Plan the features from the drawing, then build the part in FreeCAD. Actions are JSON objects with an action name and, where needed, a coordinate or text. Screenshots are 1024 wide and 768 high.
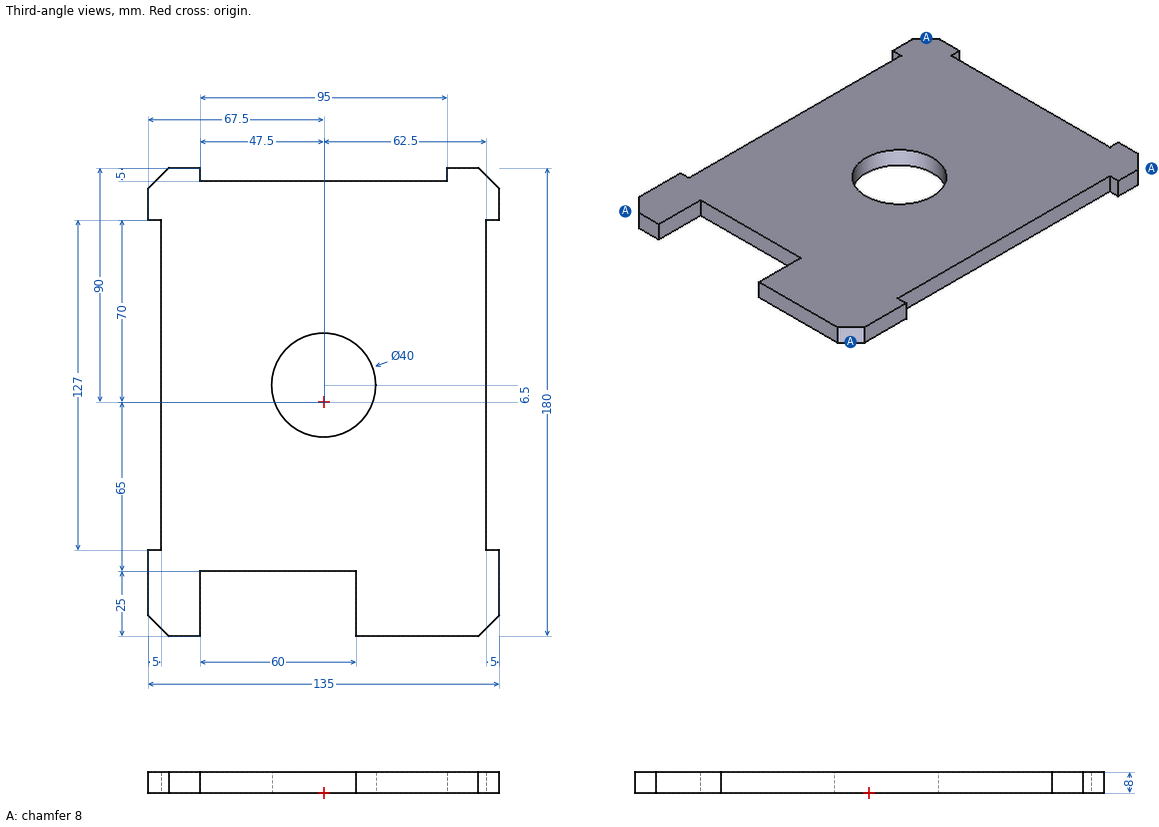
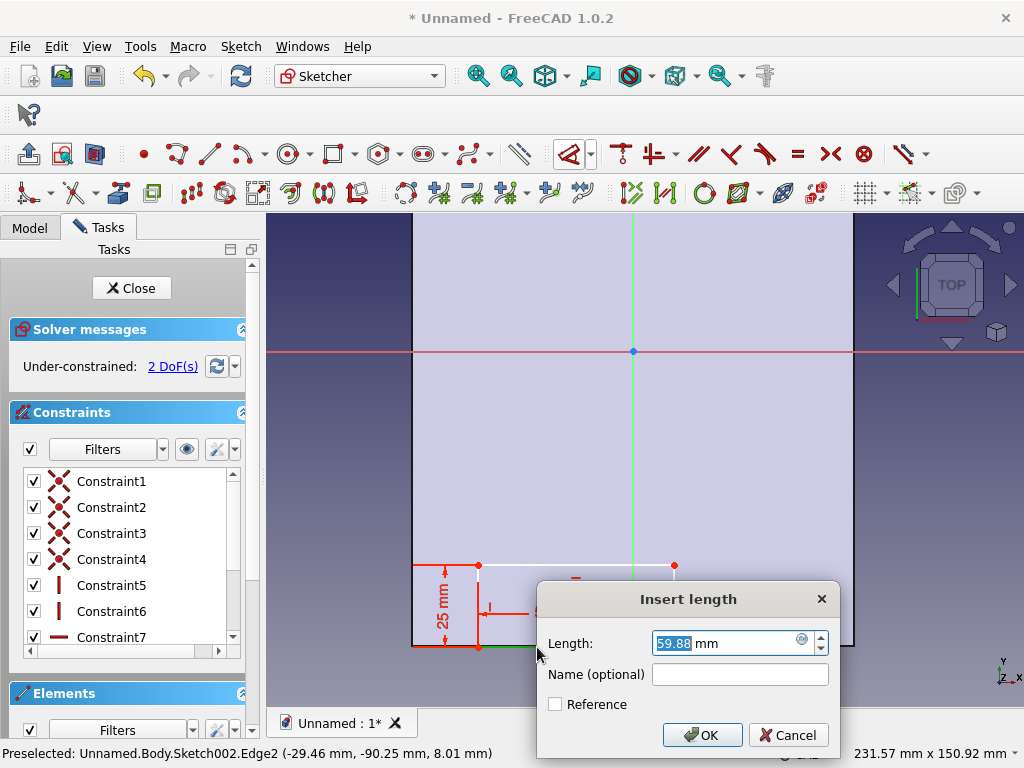
{"action": "type", "text": "60"}
{"action": "key", "text": "Return"}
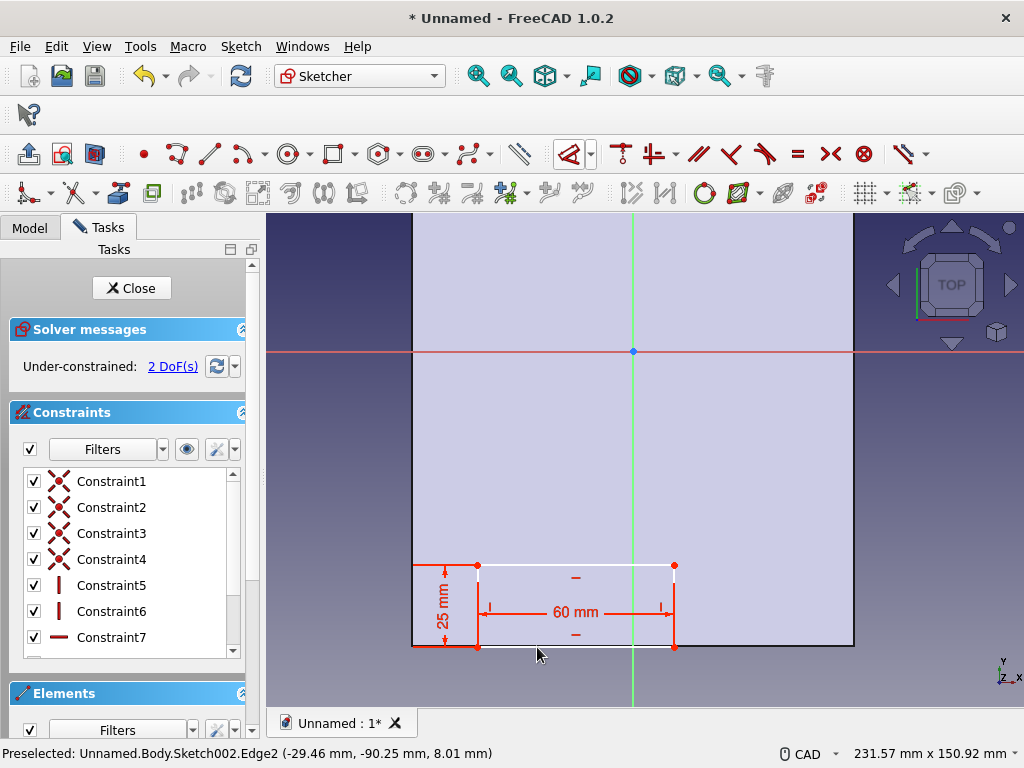
{"action": "left_click", "coordinate": [478, 565]}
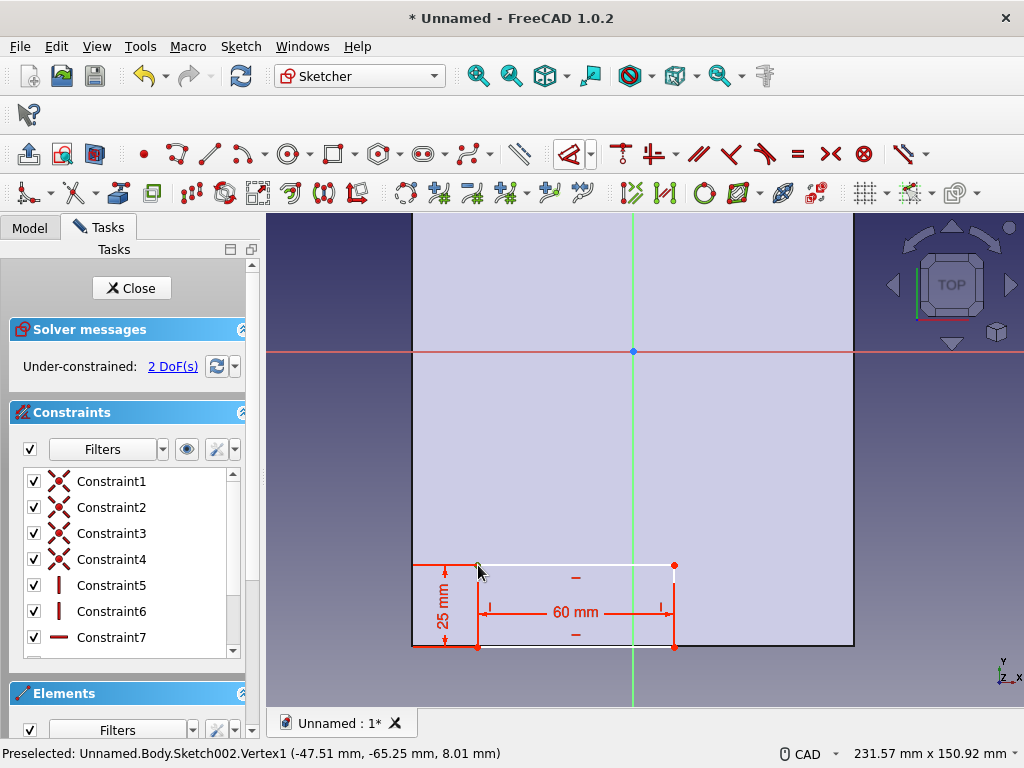
{"action": "key", "text": "i"}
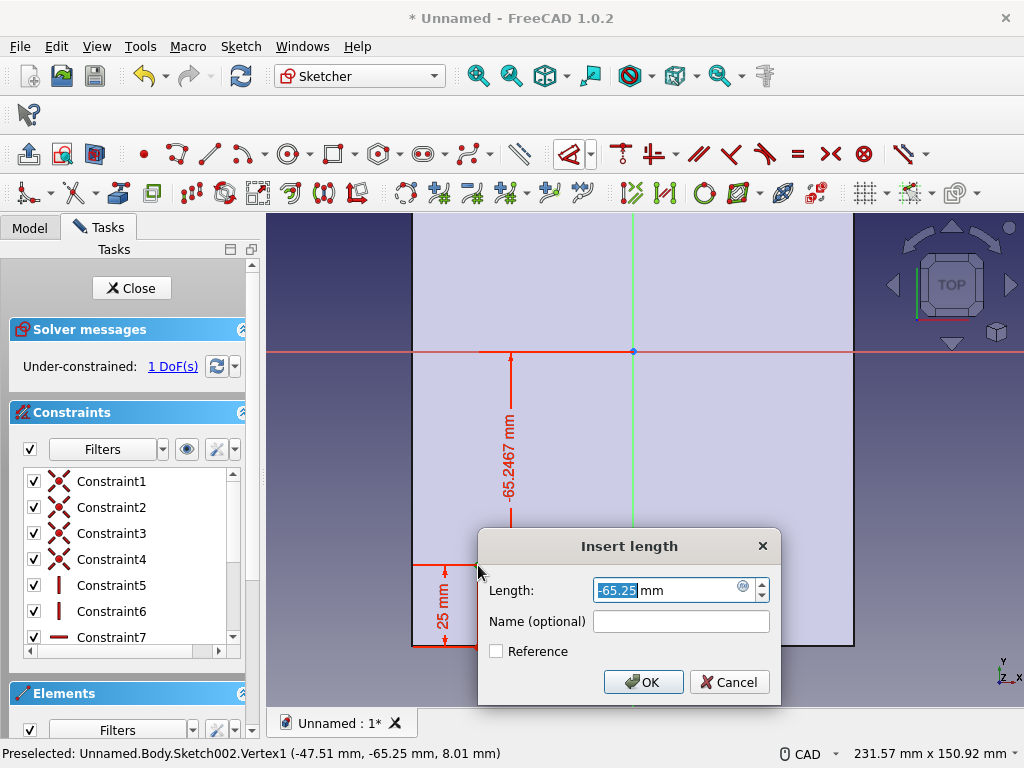
{"action": "type", "text": "-65"}
{"action": "key", "text": "Return"}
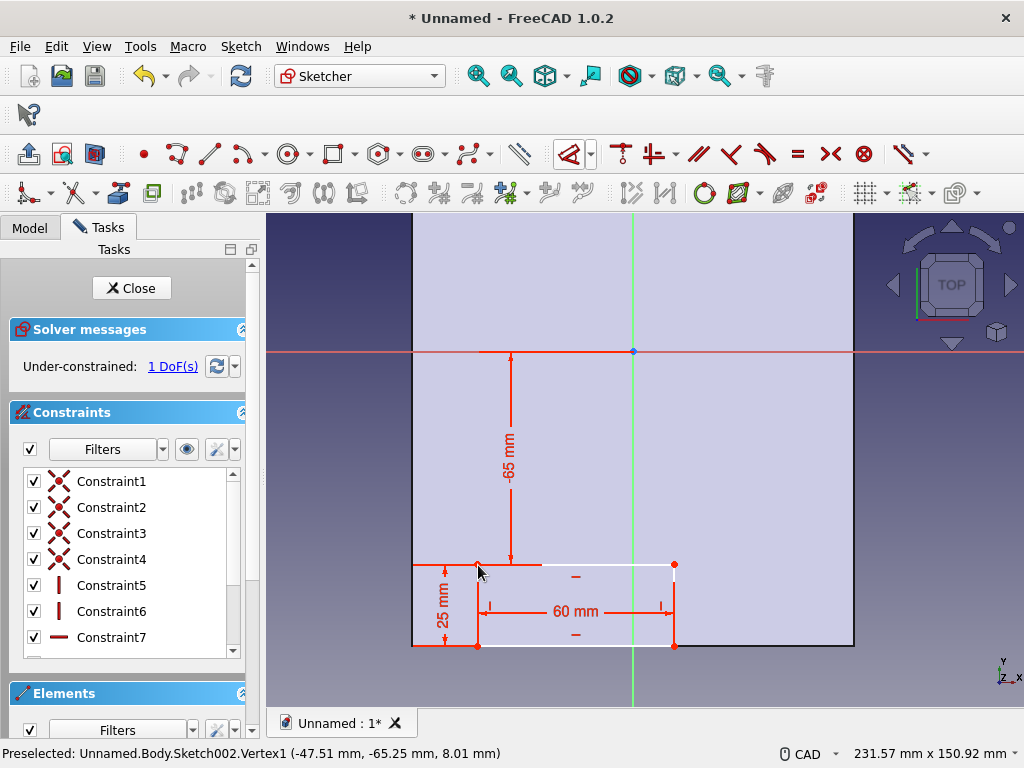
{"action": "left_click", "coordinate": [478, 565]}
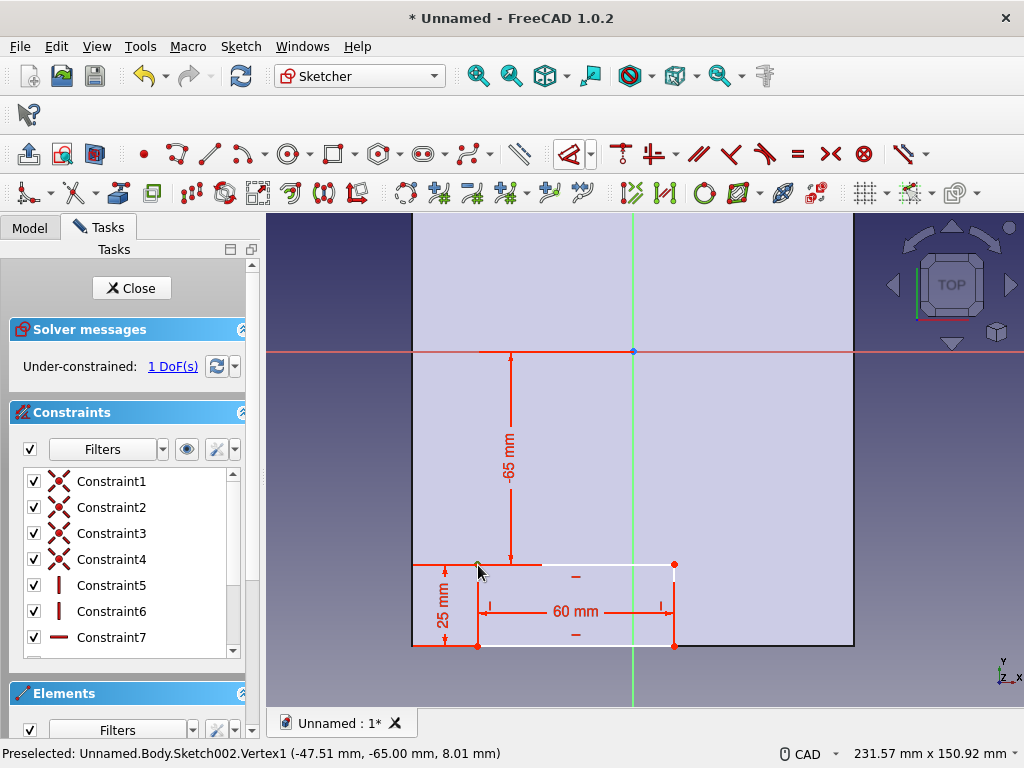
{"action": "left_click", "coordinate": [590, 154]}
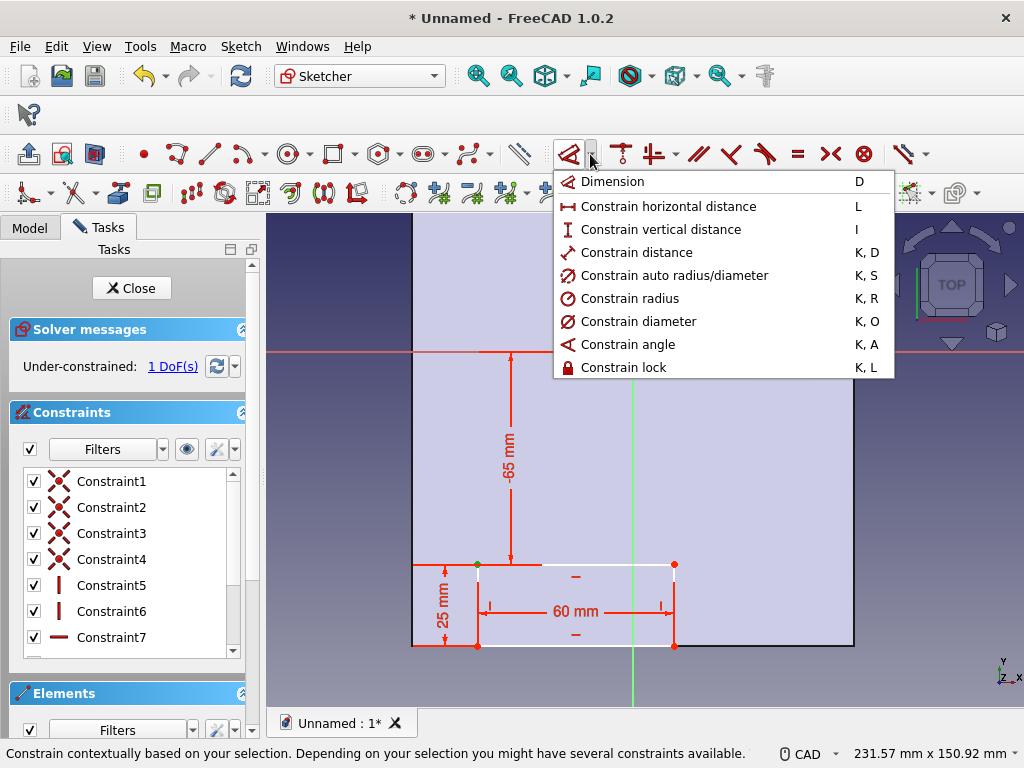
{"action": "left_click", "coordinate": [724, 206]}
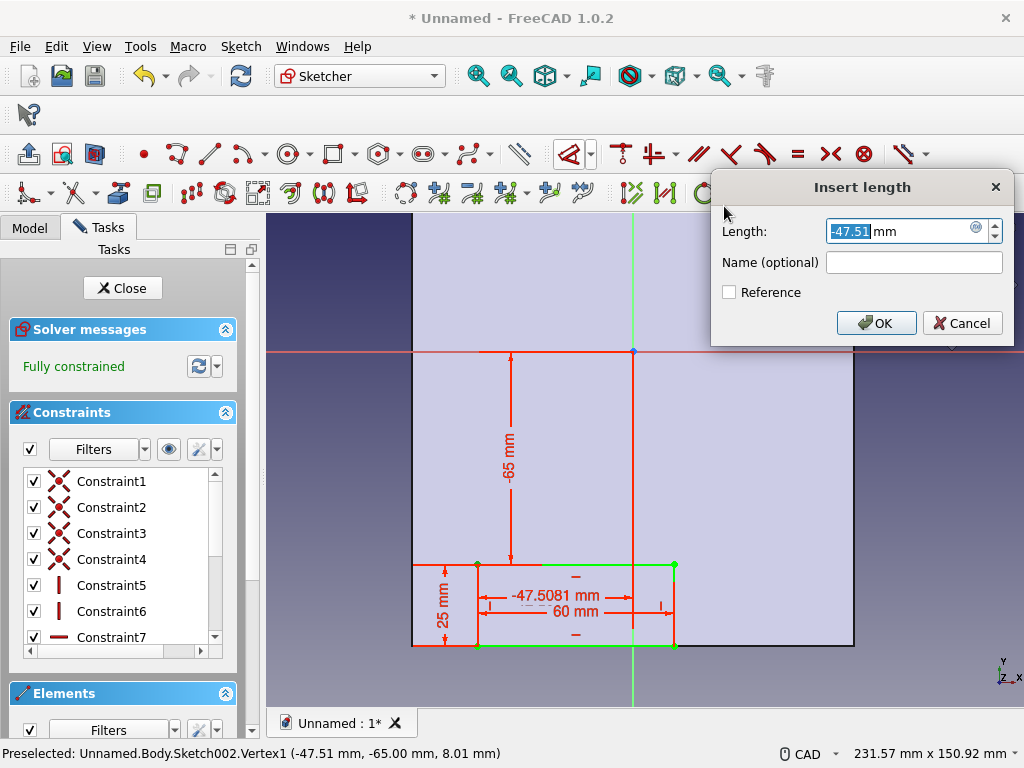
{"action": "type", "text": "-47.5"}
{"action": "key", "text": "Return"}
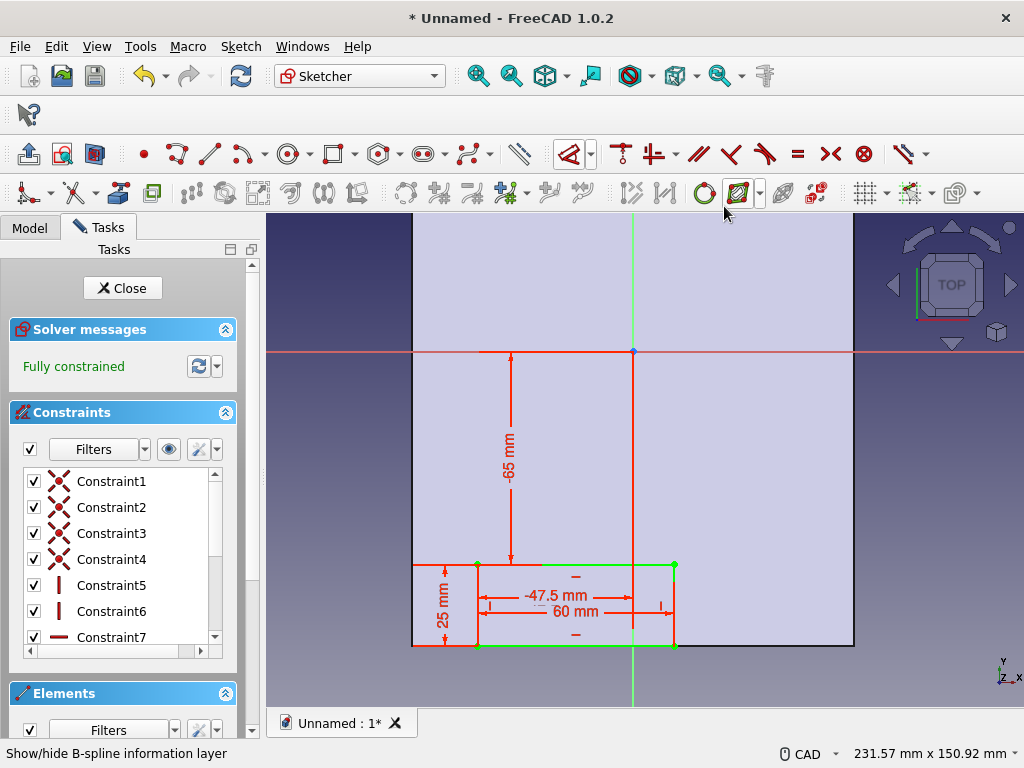
{"action": "left_click", "coordinate": [123, 288]}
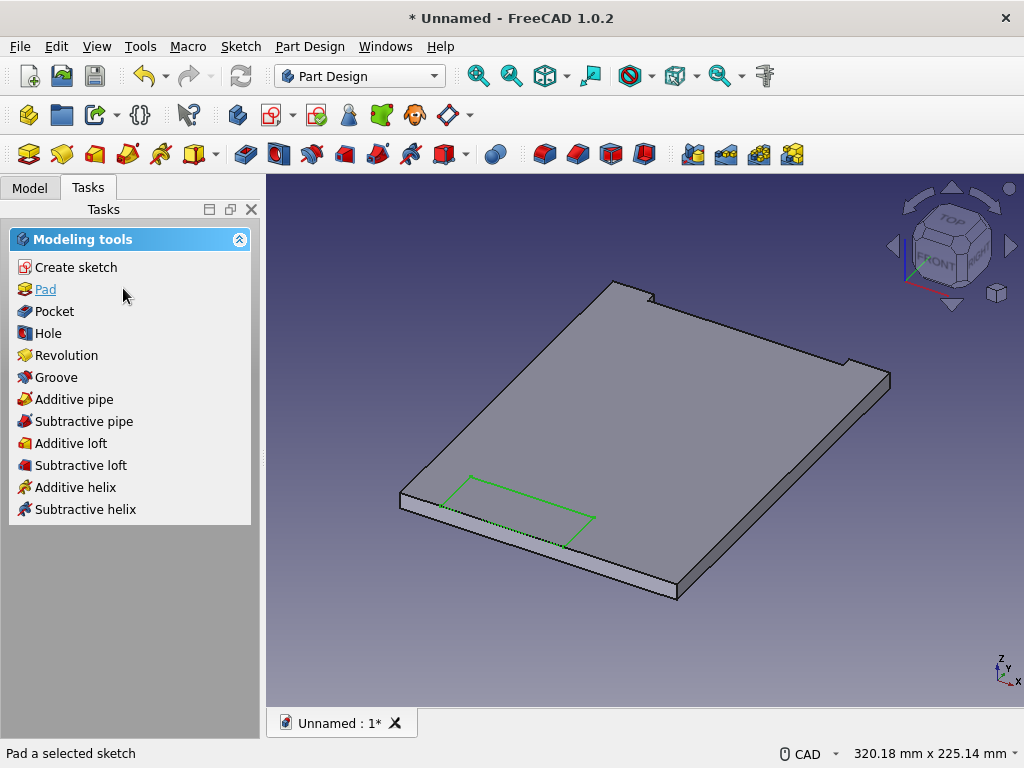
{"action": "left_click", "coordinate": [246, 154]}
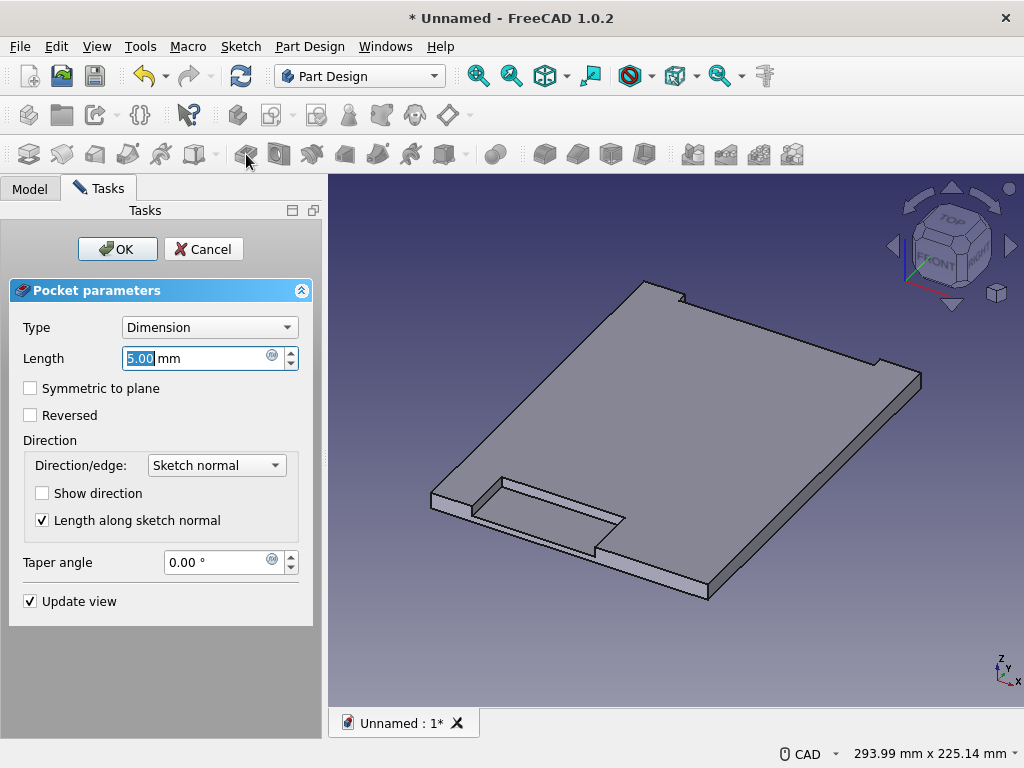
{"action": "left_click", "coordinate": [210, 328]}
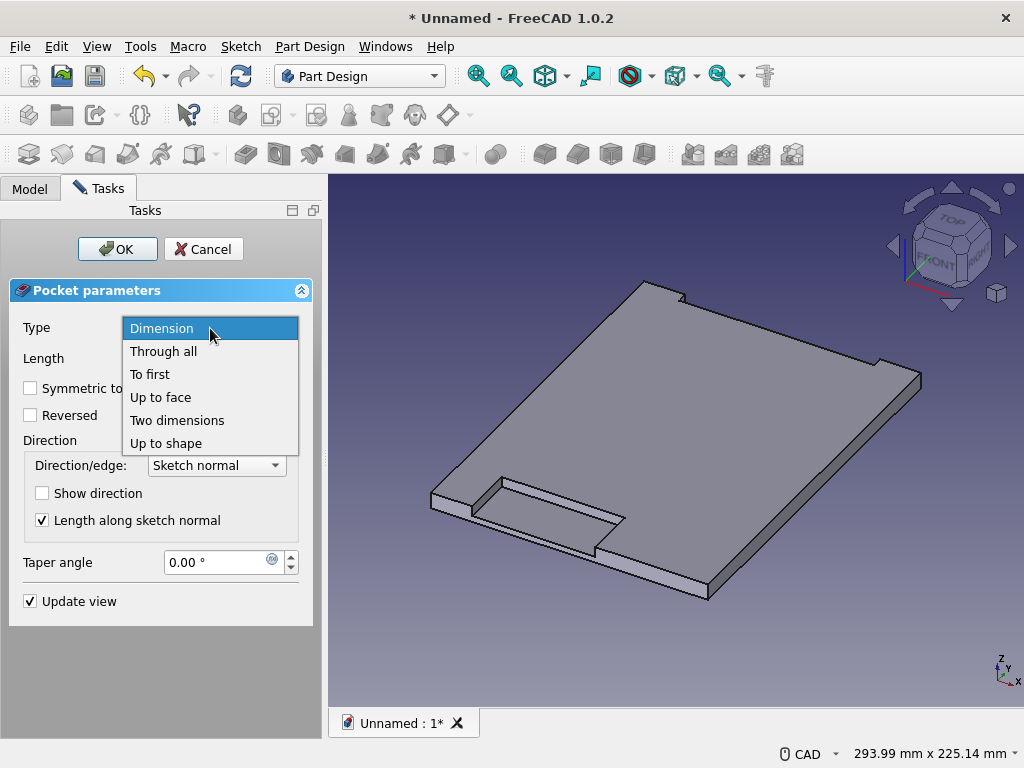
{"action": "left_click", "coordinate": [208, 374]}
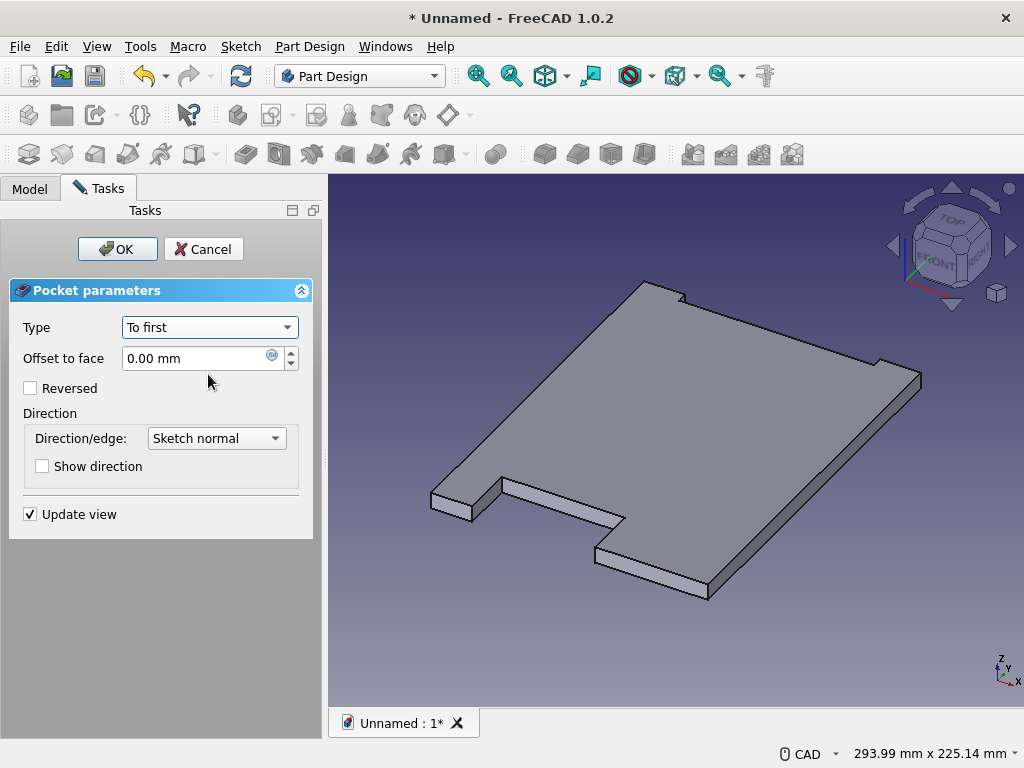
{"action": "left_click", "coordinate": [118, 249]}